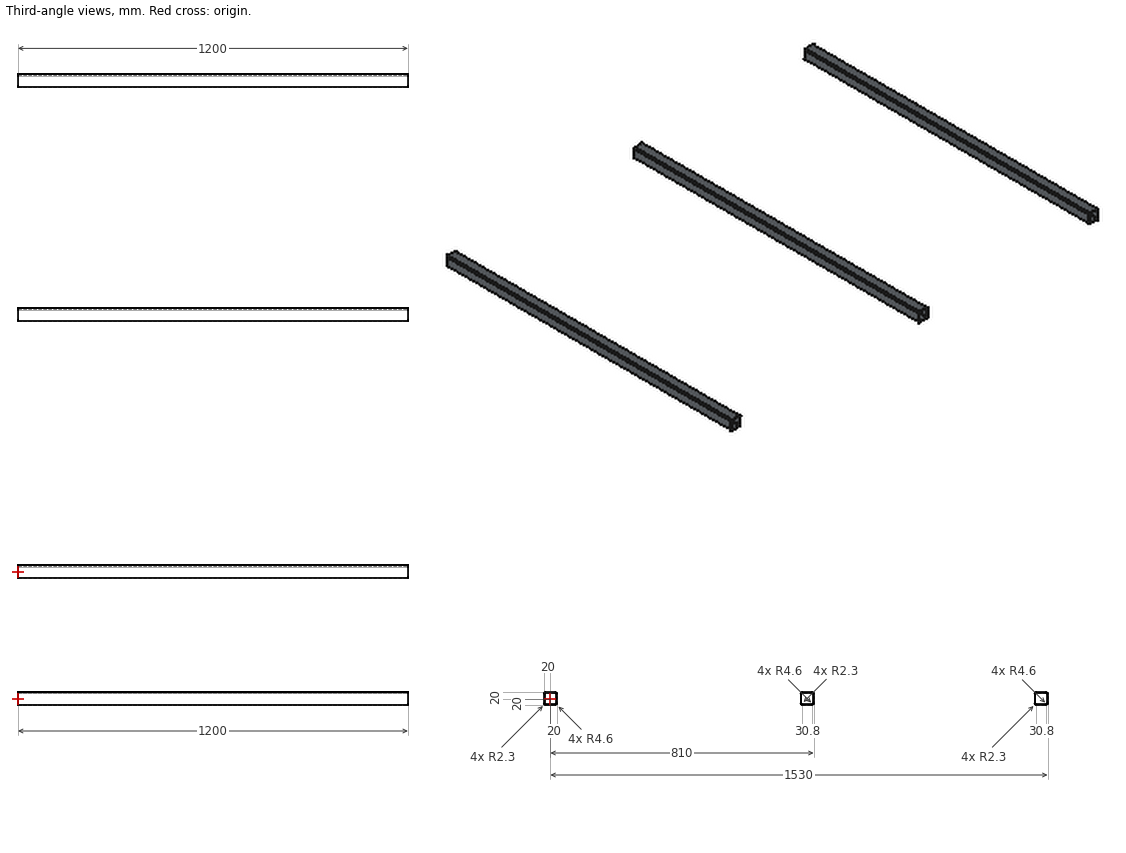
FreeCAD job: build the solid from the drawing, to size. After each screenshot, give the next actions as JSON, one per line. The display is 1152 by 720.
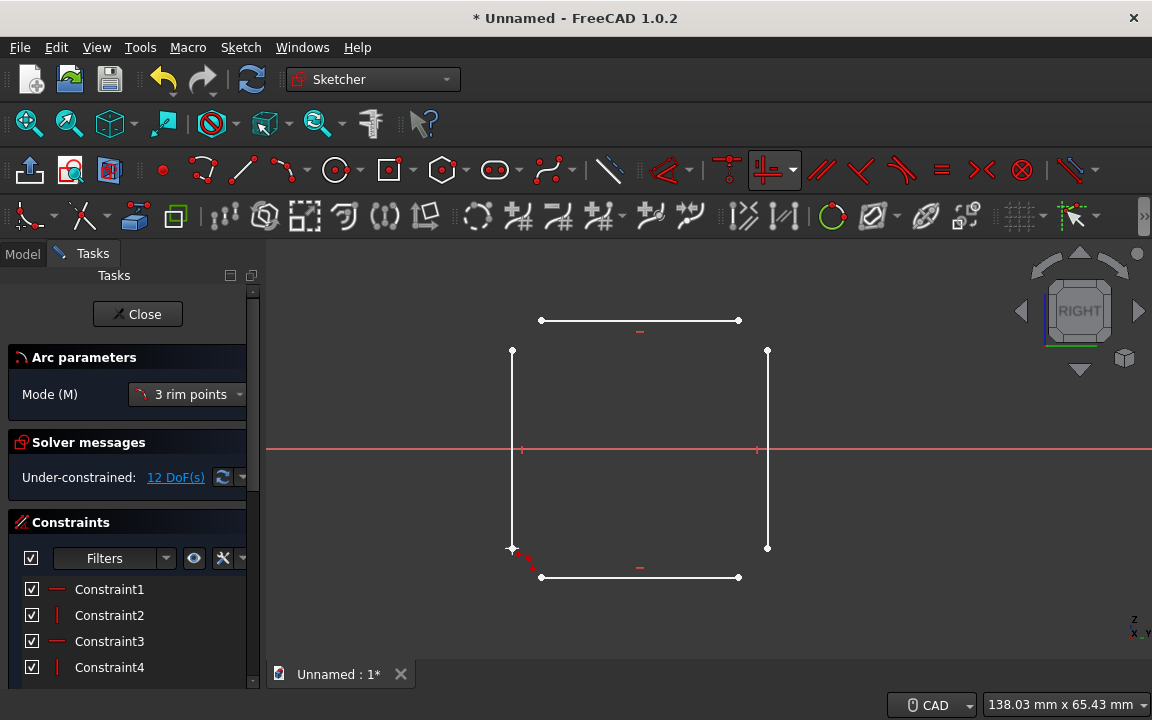
{"action": "left_click", "coordinate": [739, 578]}
{"action": "left_click", "coordinate": [768, 549]}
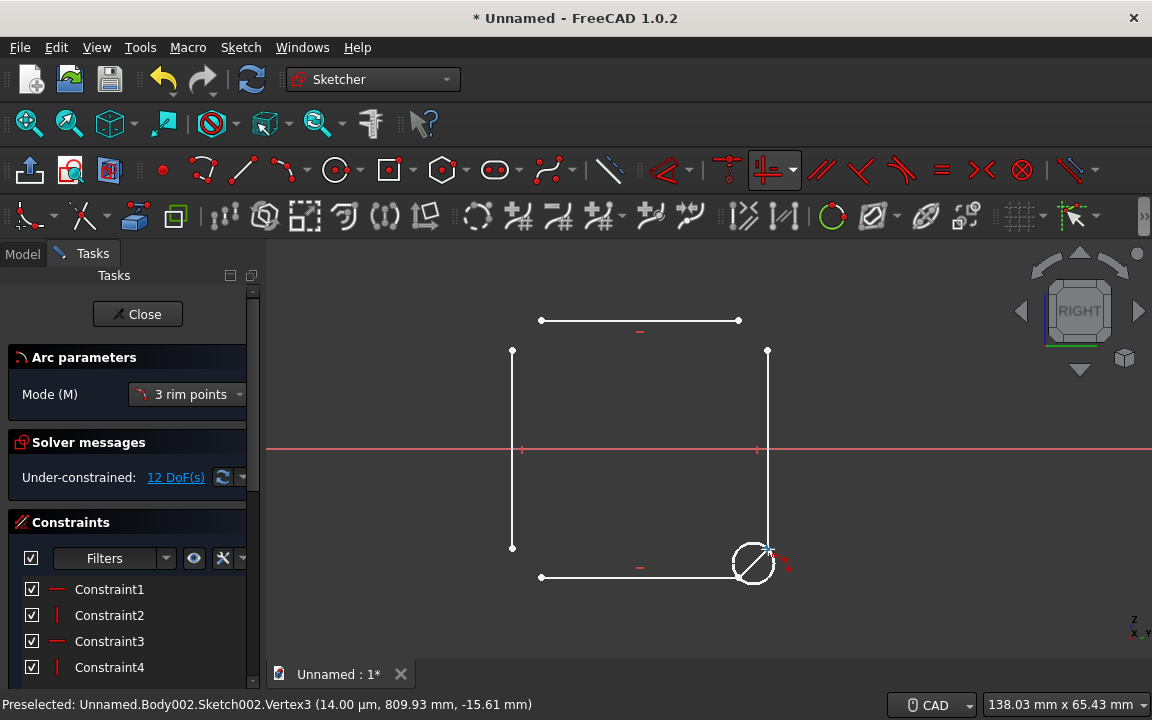
{"action": "scroll", "coordinate": [760, 569], "scroll_direction": "up", "scroll_amount": 4}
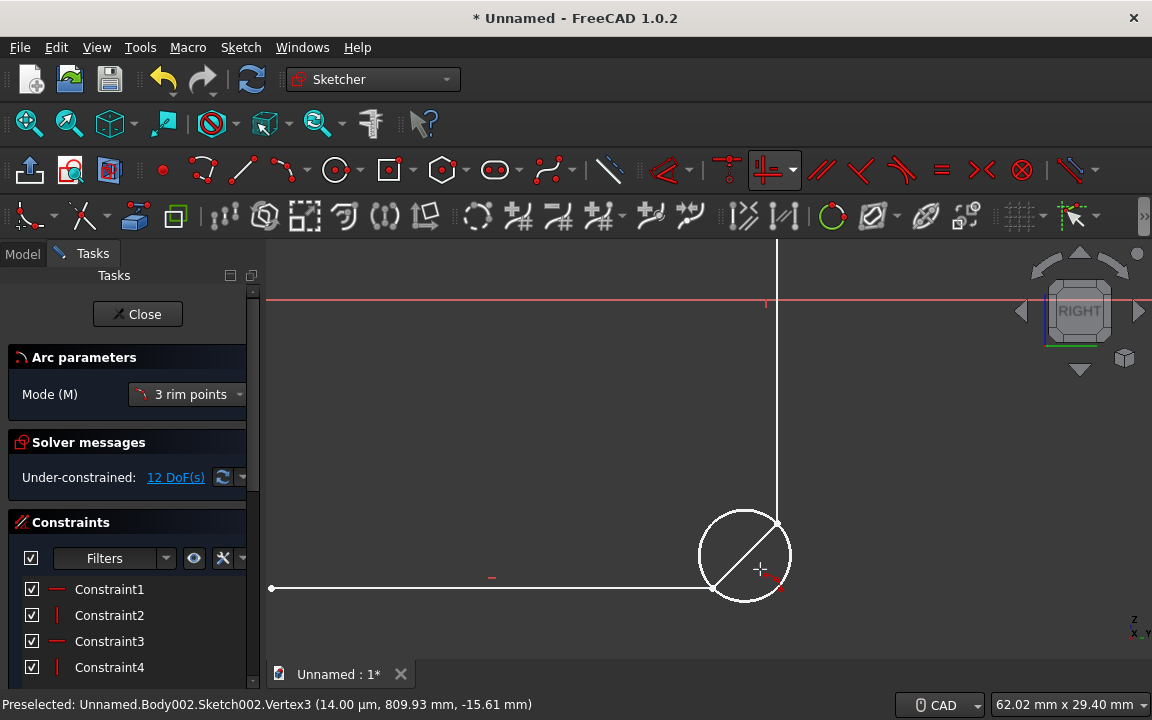
{"action": "left_click", "coordinate": [759, 567]}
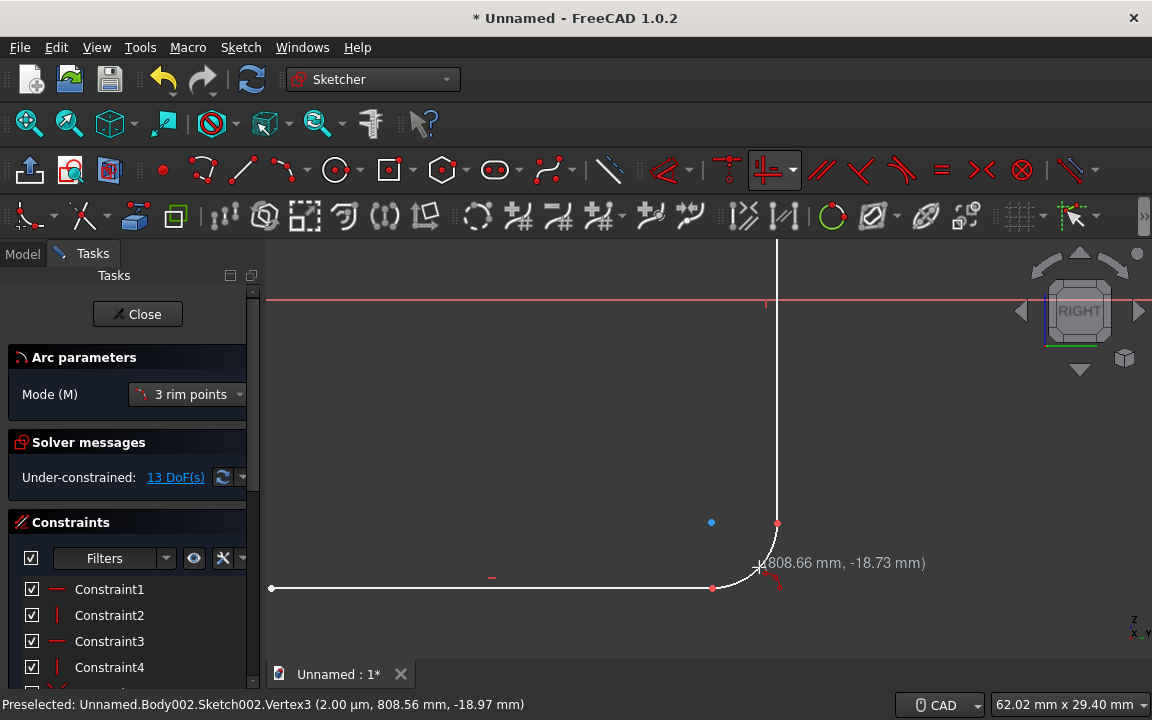
{"action": "scroll", "coordinate": [761, 570], "scroll_direction": "down", "scroll_amount": 4}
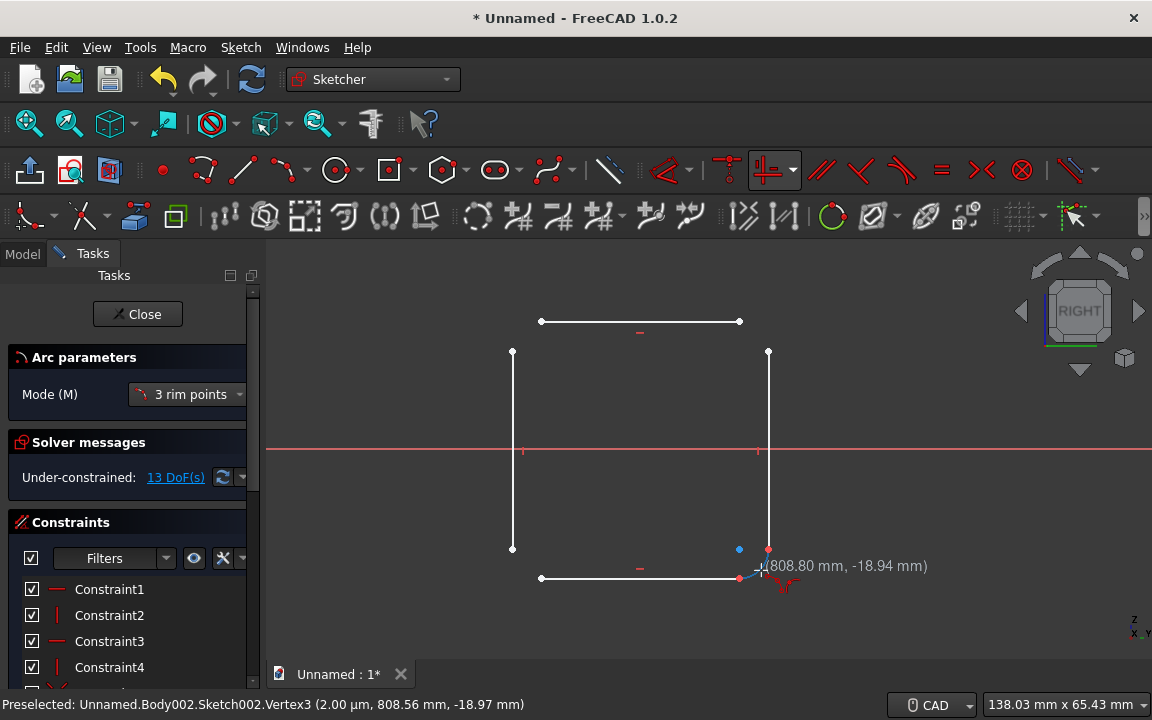
{"action": "left_click", "coordinate": [769, 352]}
{"action": "left_click", "coordinate": [740, 322]}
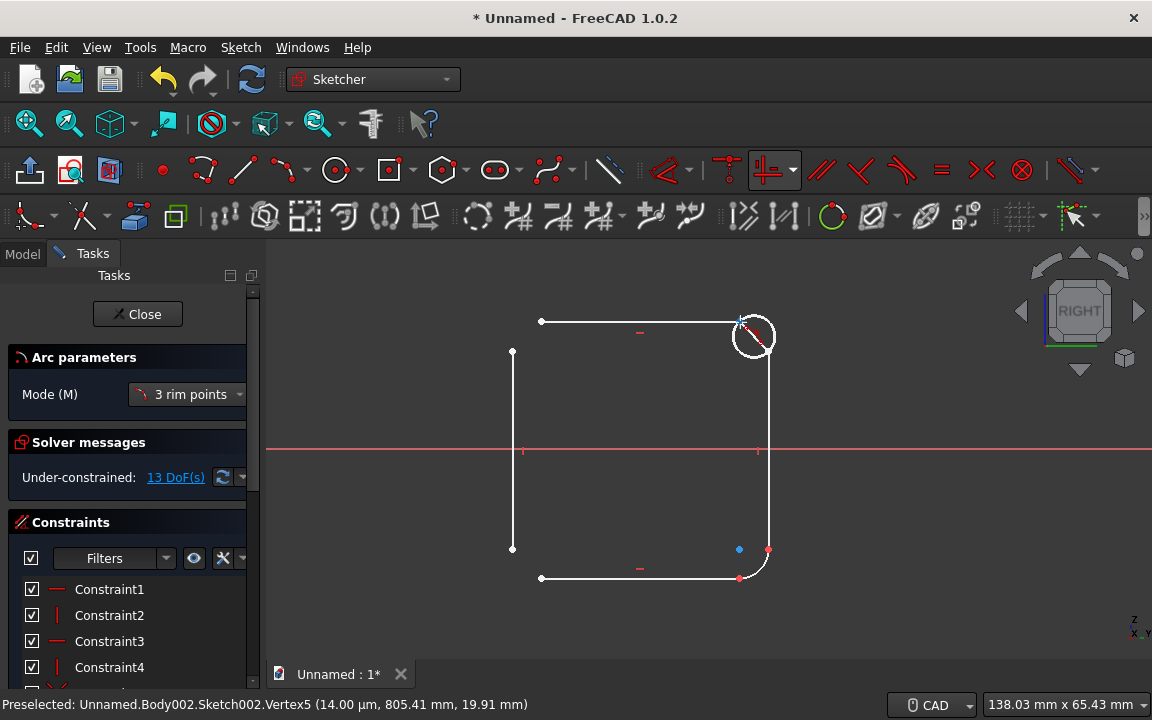
{"action": "scroll", "coordinate": [760, 330], "scroll_direction": "up", "scroll_amount": 4}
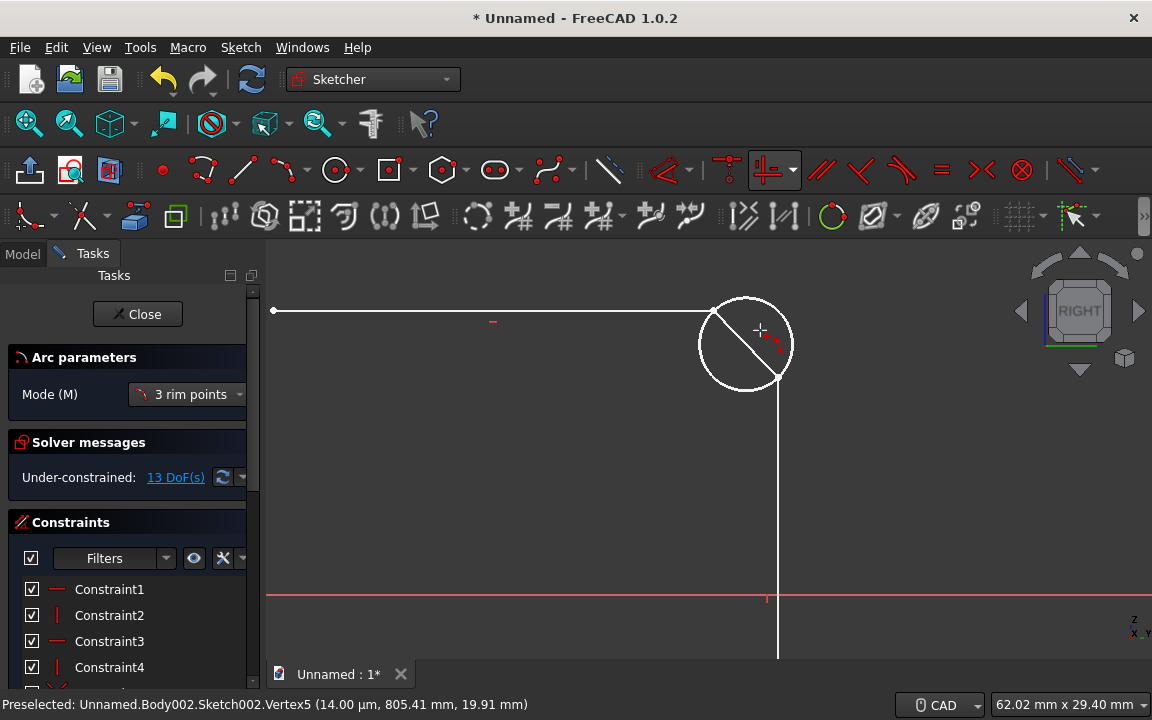
{"action": "left_click", "coordinate": [760, 329]}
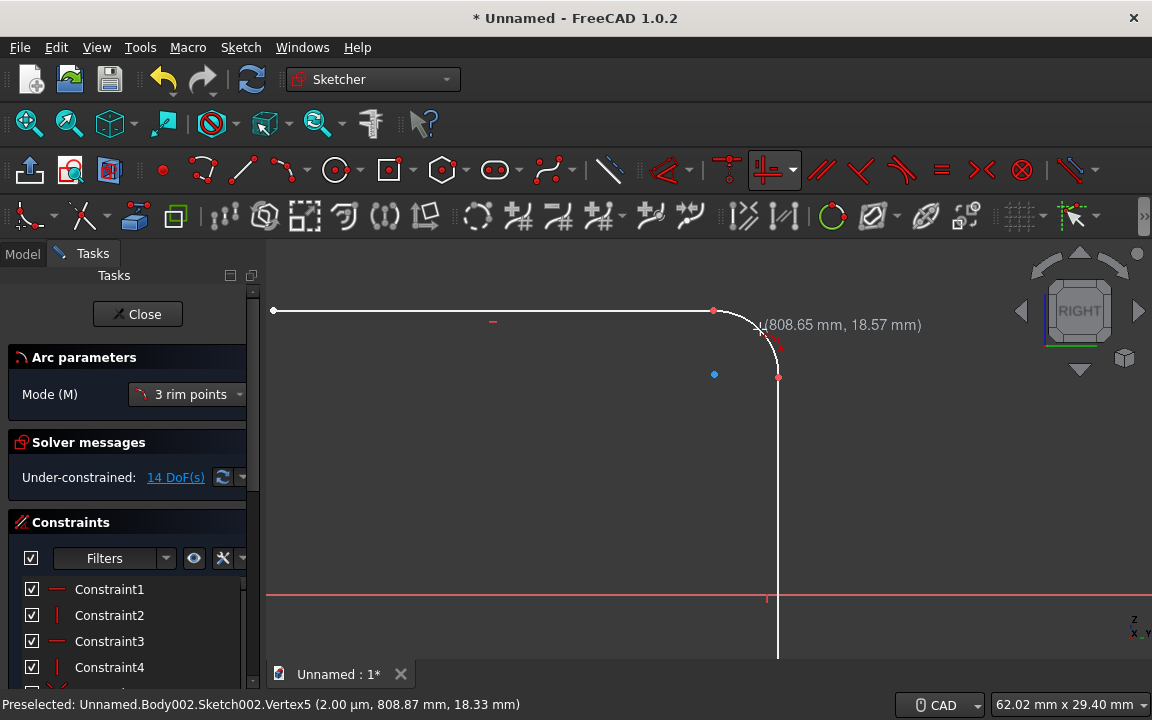
{"action": "scroll", "coordinate": [760, 330], "scroll_direction": "down", "scroll_amount": 4}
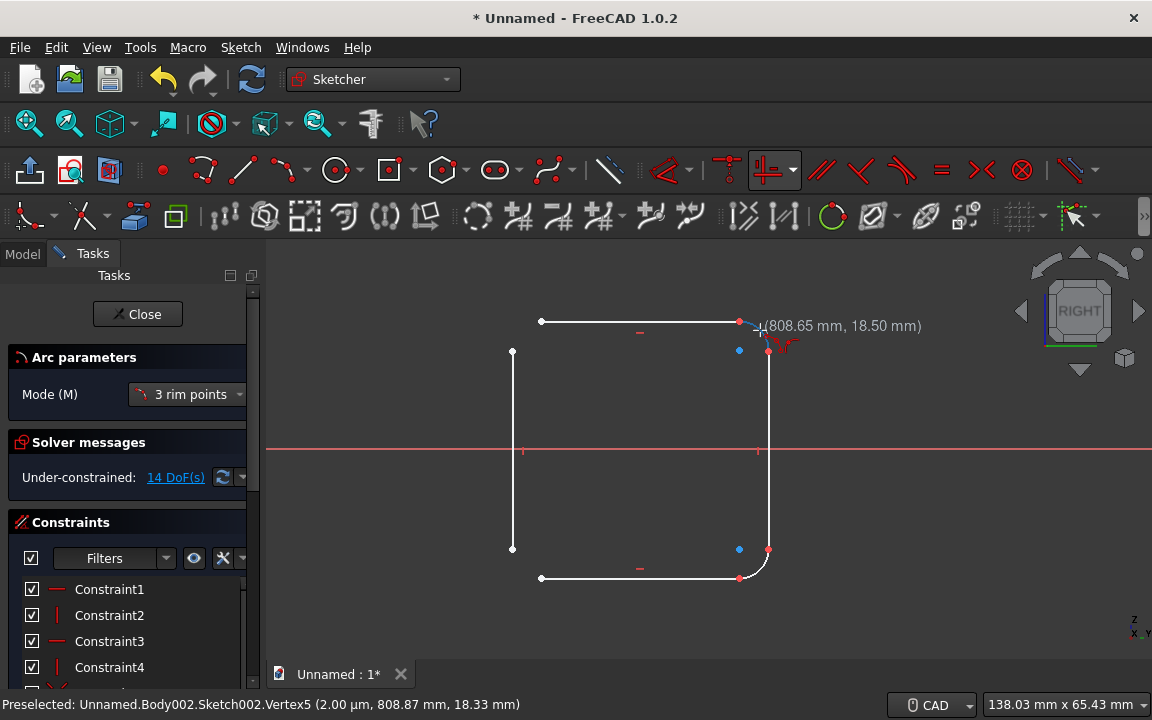
{"action": "left_click", "coordinate": [542, 322]}
{"action": "left_click", "coordinate": [513, 352]}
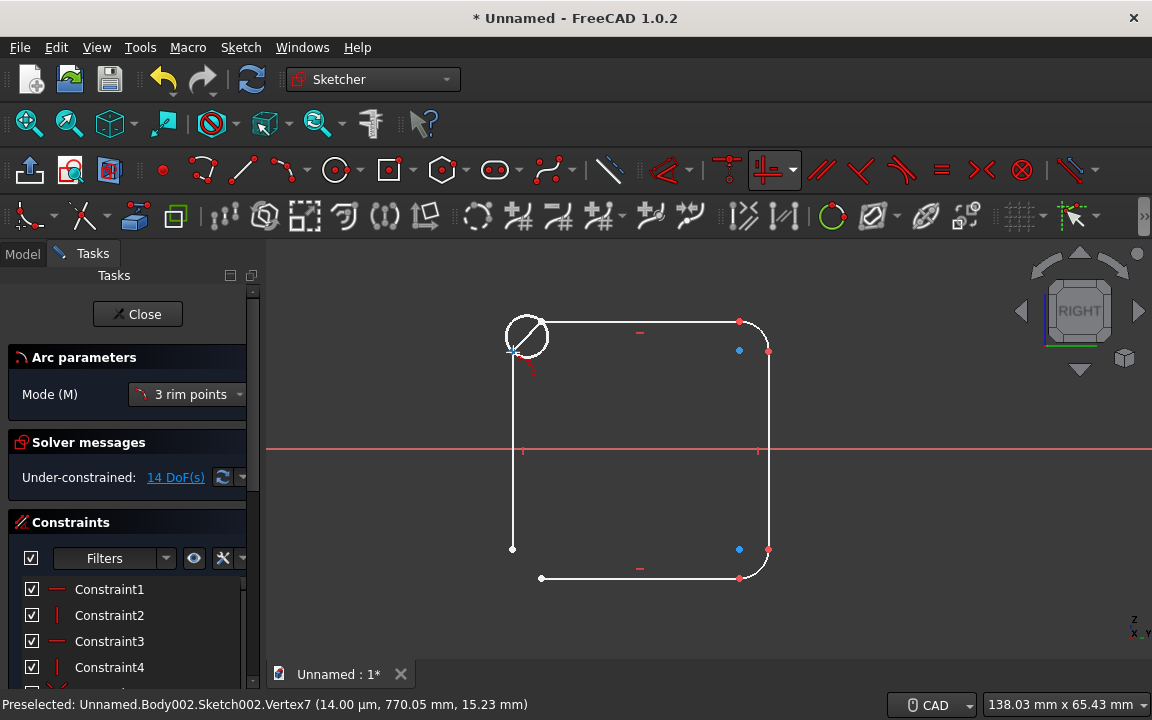
{"action": "scroll", "coordinate": [521, 330], "scroll_direction": "up", "scroll_amount": 4}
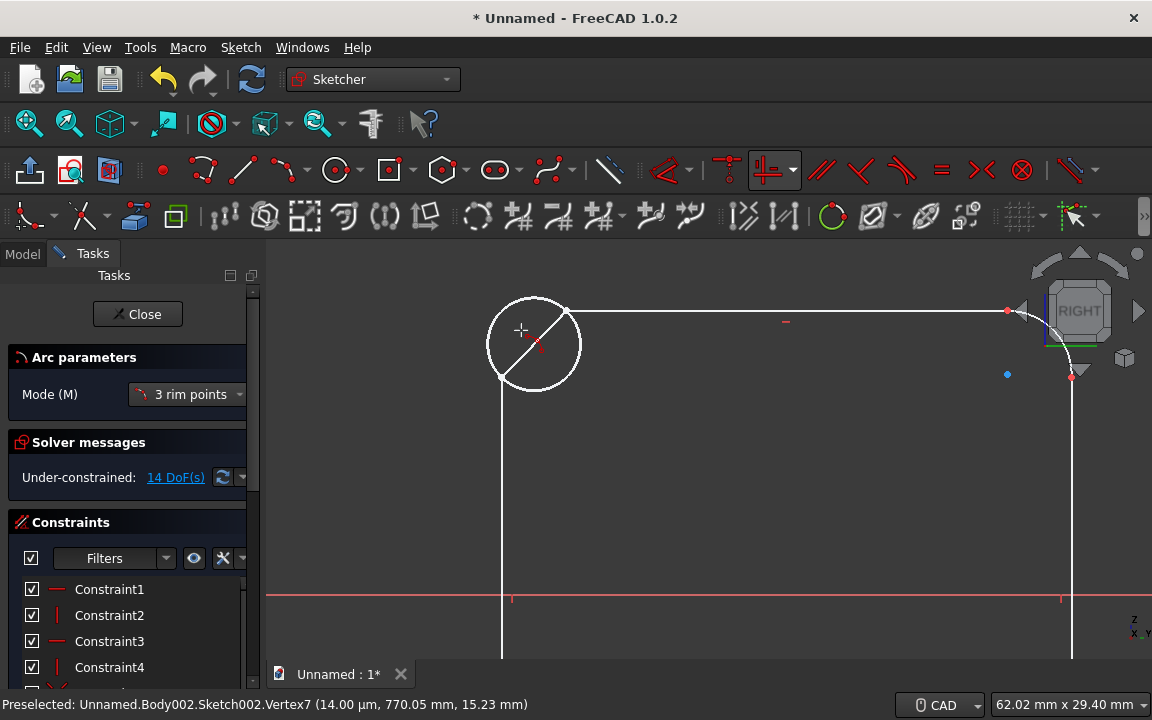
{"action": "left_click", "coordinate": [520, 329]}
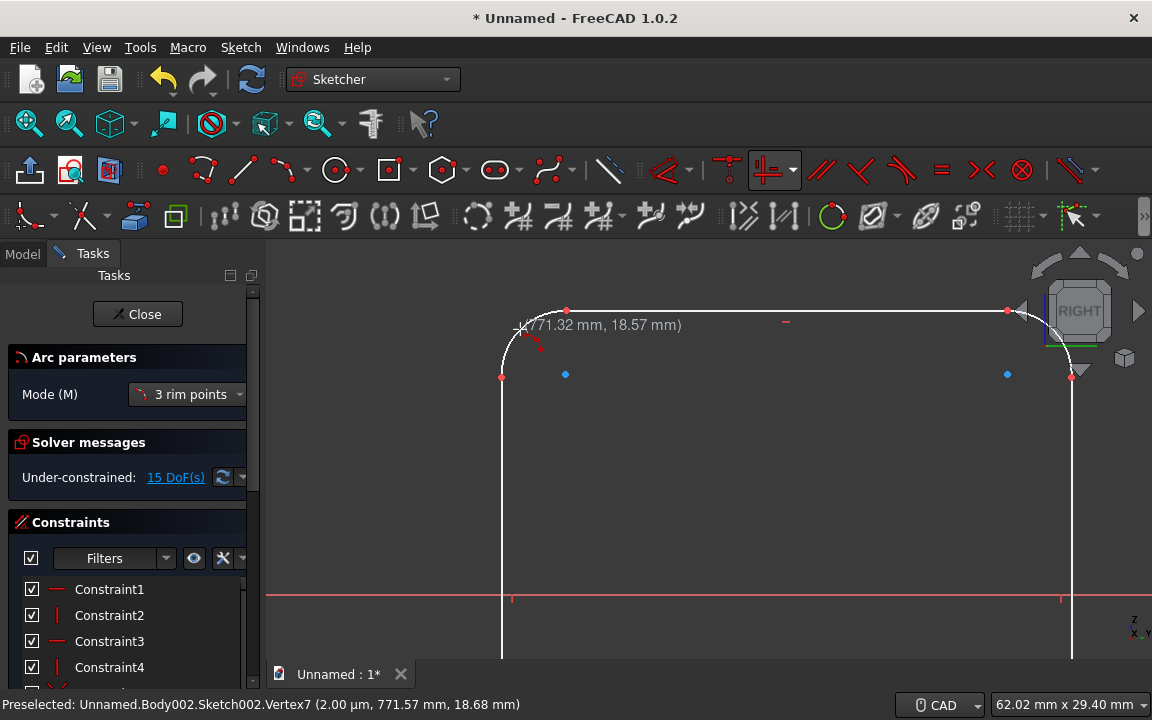
{"action": "scroll", "coordinate": [521, 330], "scroll_direction": "down", "scroll_amount": 4}